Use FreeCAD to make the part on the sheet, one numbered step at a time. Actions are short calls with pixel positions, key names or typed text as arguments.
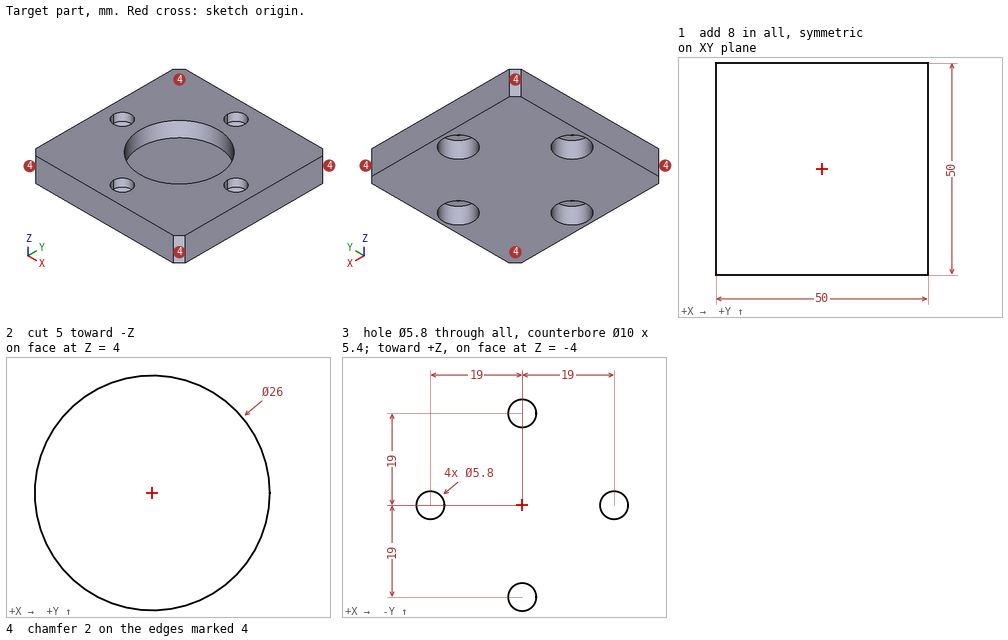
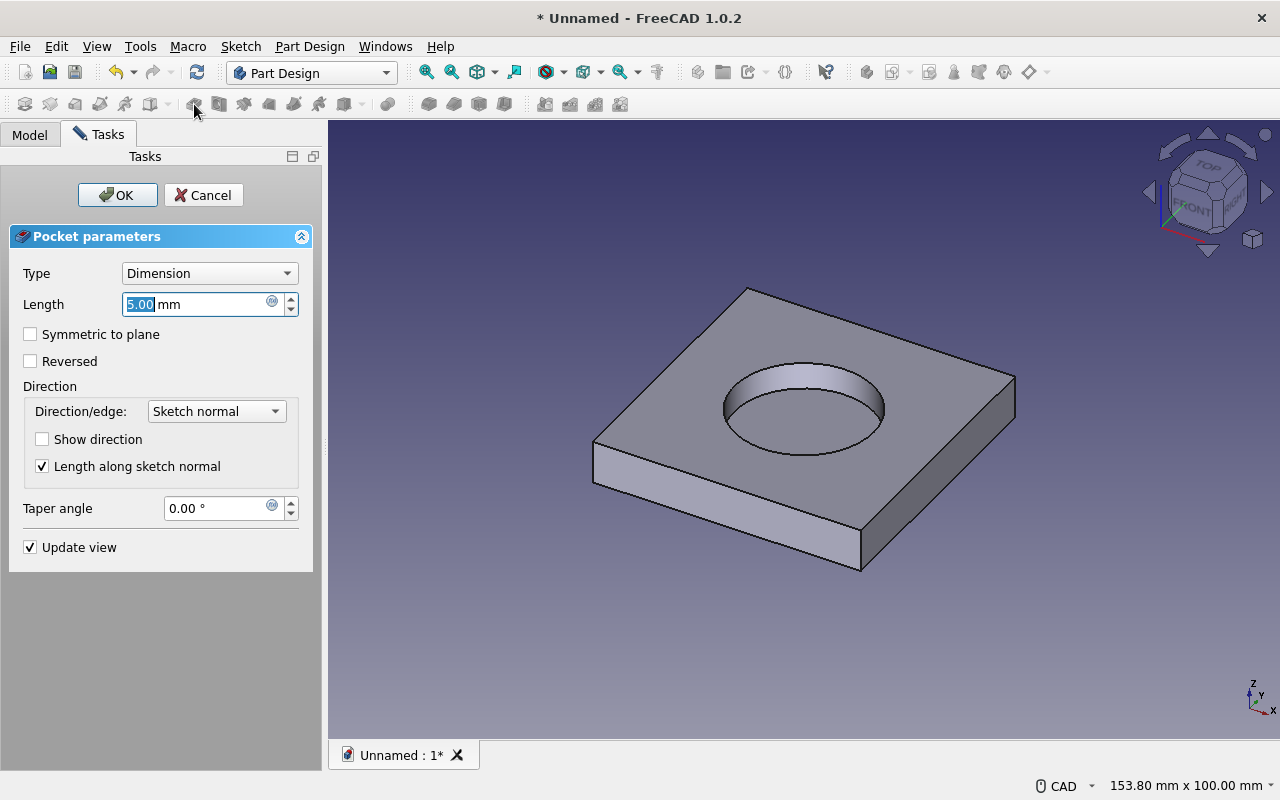
text(5)
key(Tab)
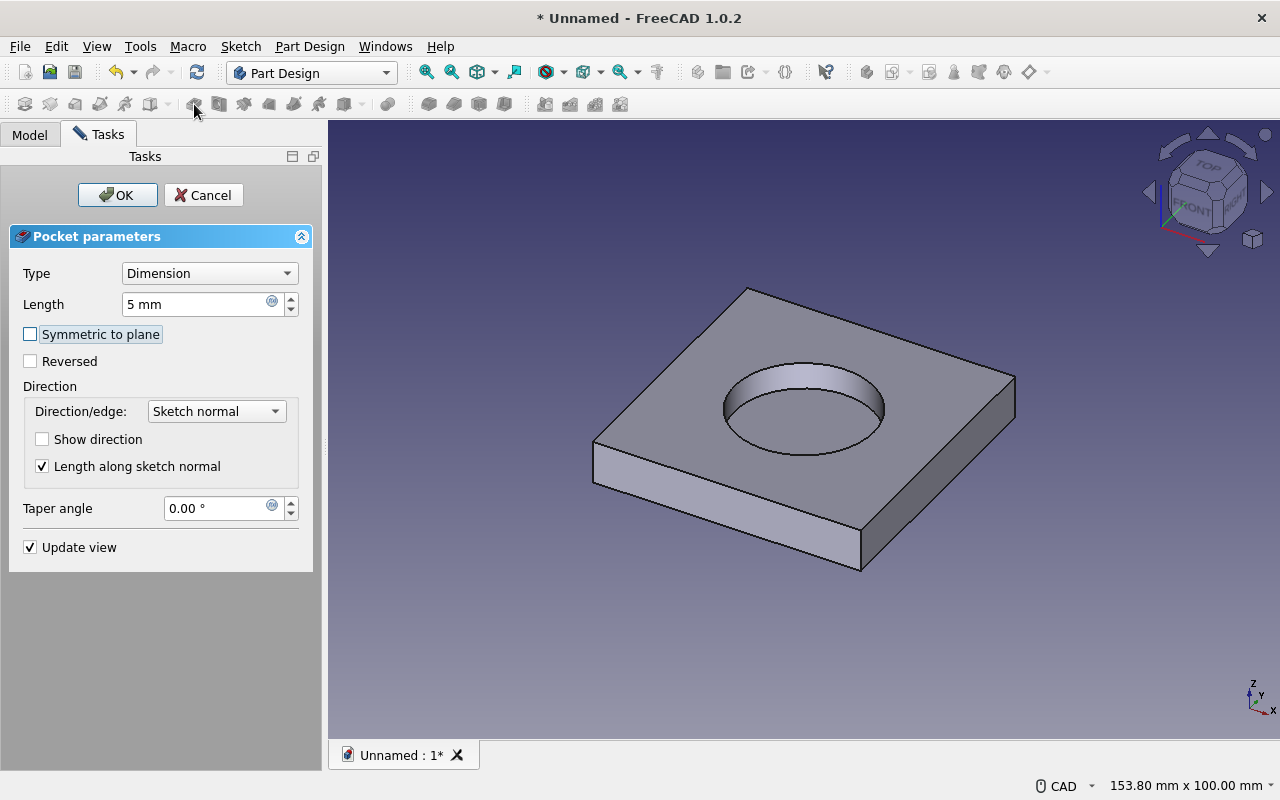
click(118, 195)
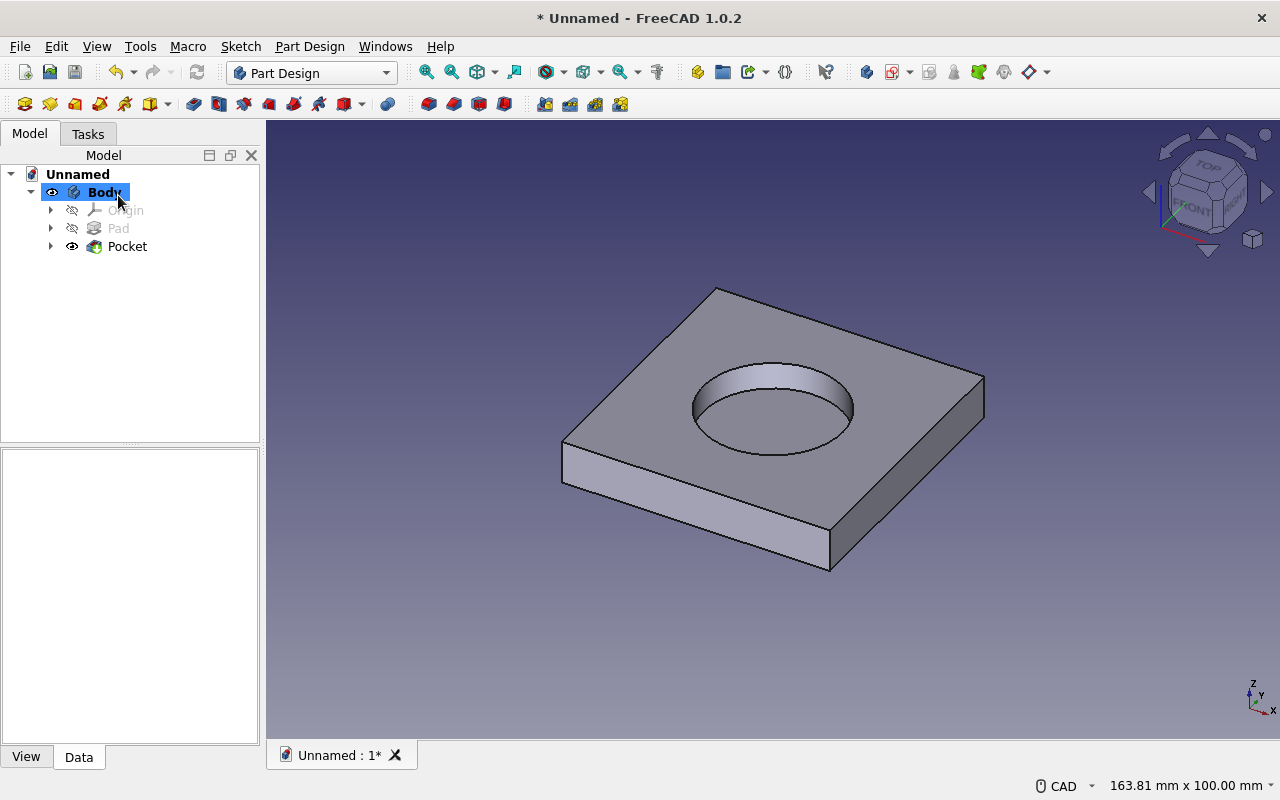
key(5)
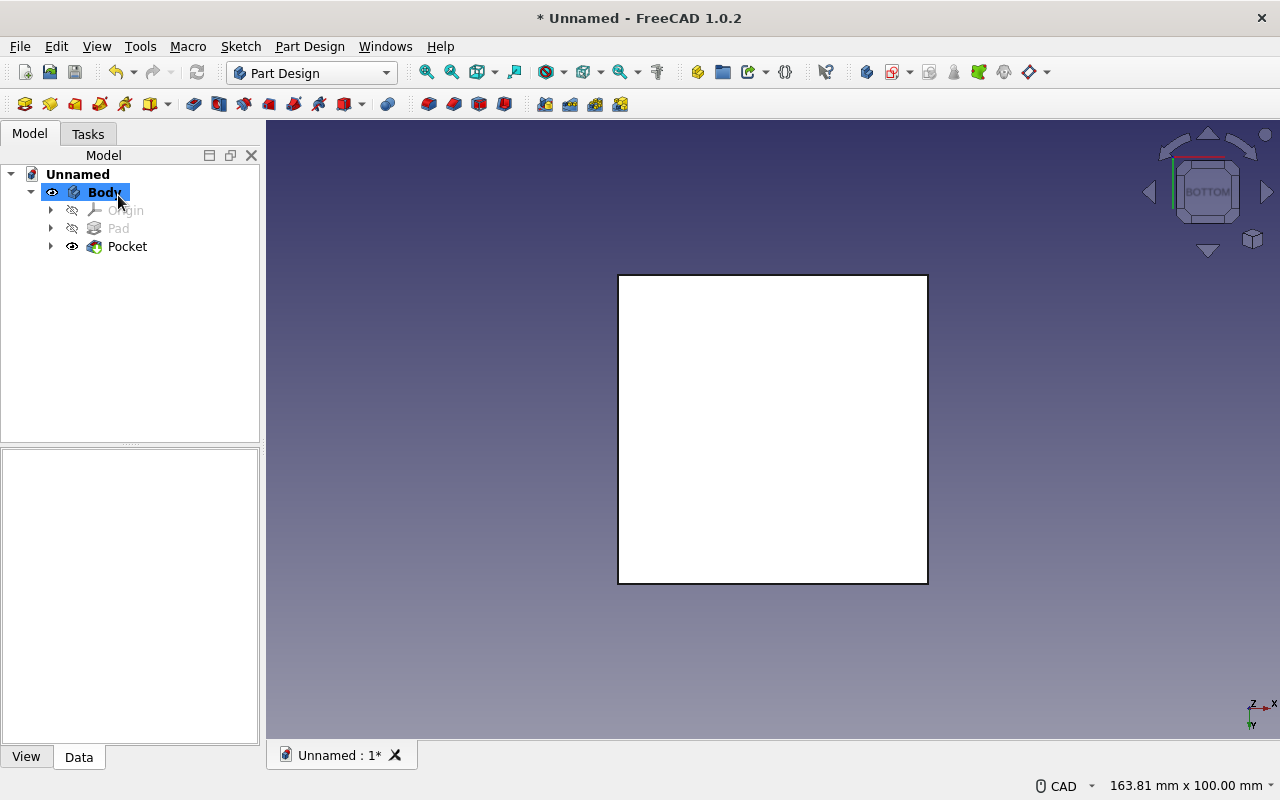
click(773, 428)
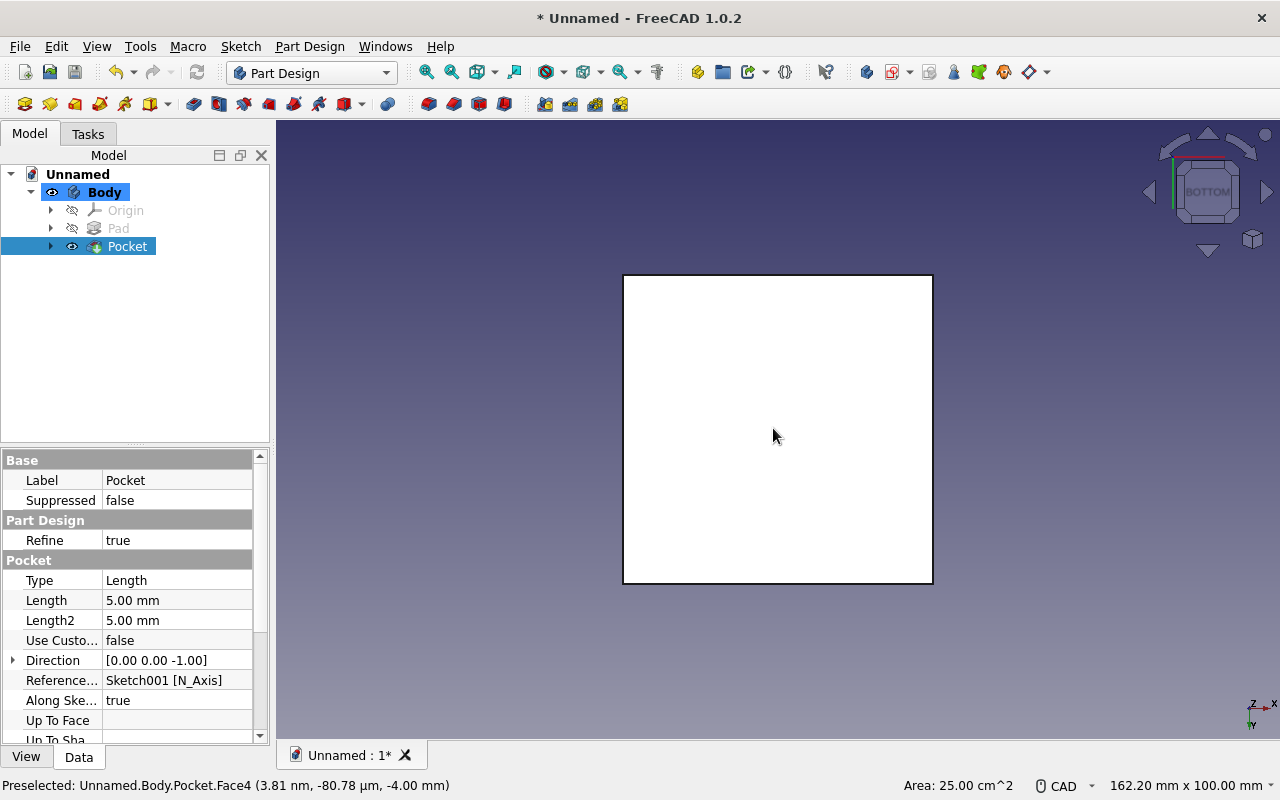
click(892, 72)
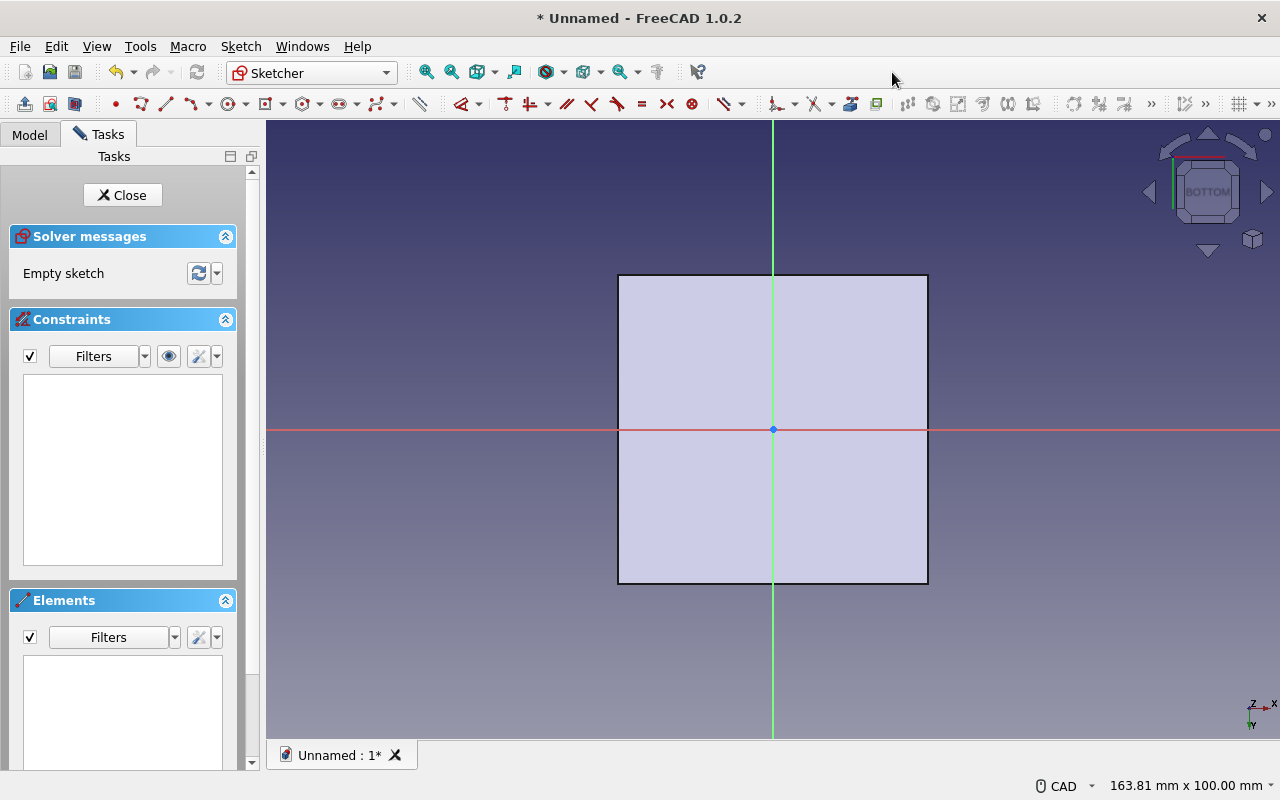
scroll(912, 429, up, 2)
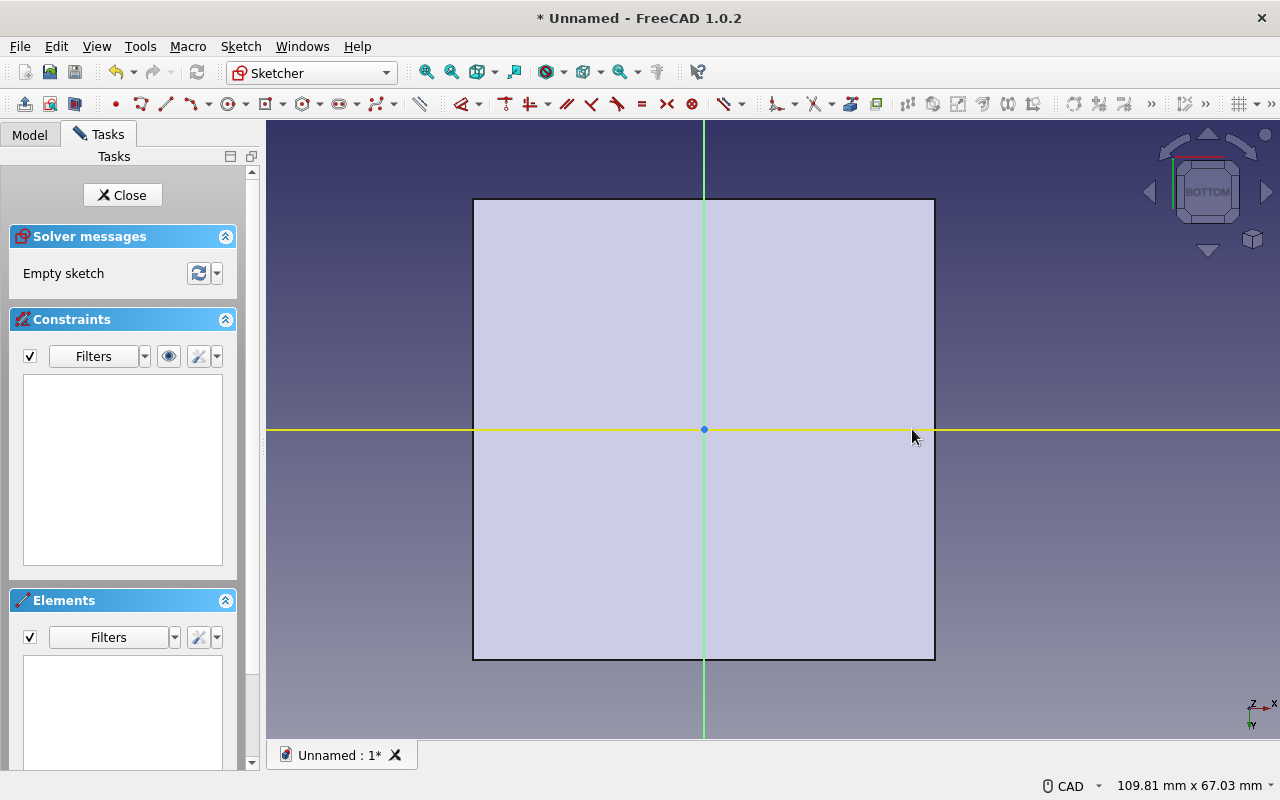
click(228, 104)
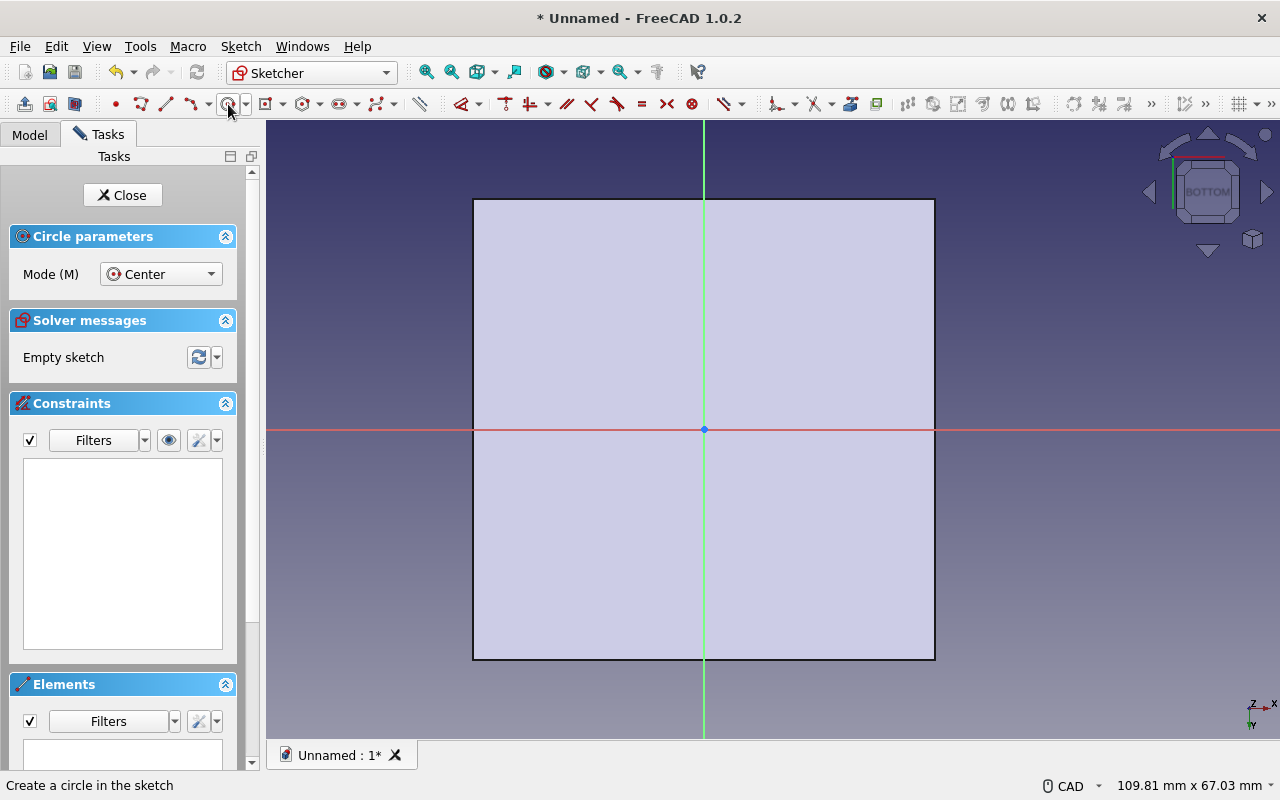
click(529, 430)
move(548, 411)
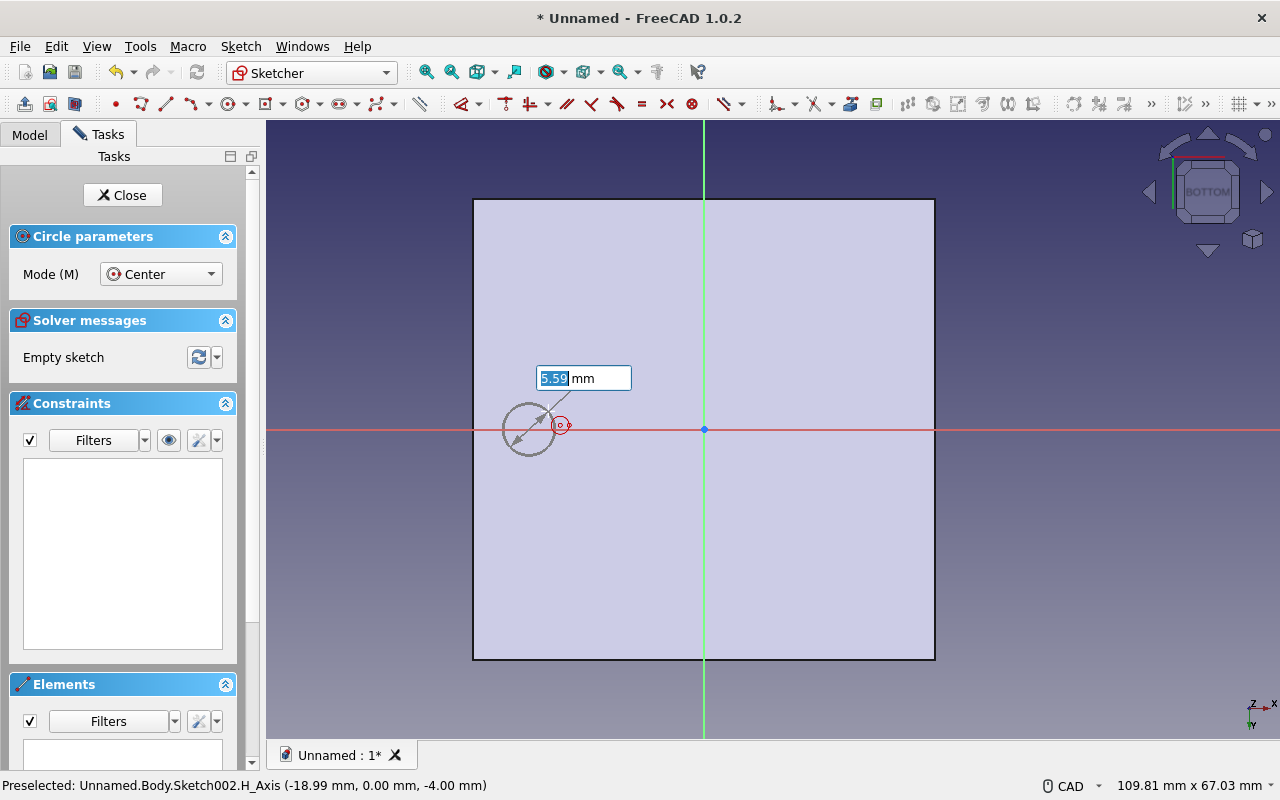
text(5.8)
key(Return)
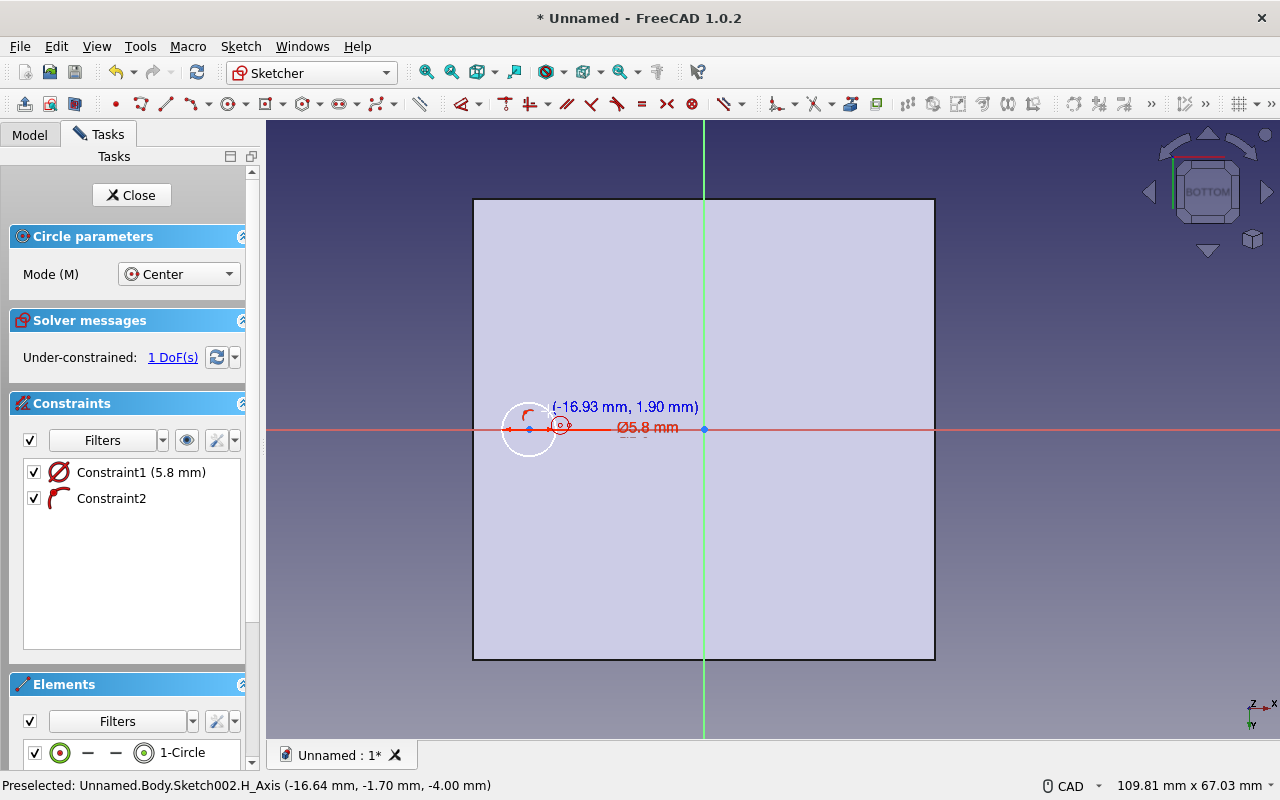
click(704, 605)
move(723, 586)